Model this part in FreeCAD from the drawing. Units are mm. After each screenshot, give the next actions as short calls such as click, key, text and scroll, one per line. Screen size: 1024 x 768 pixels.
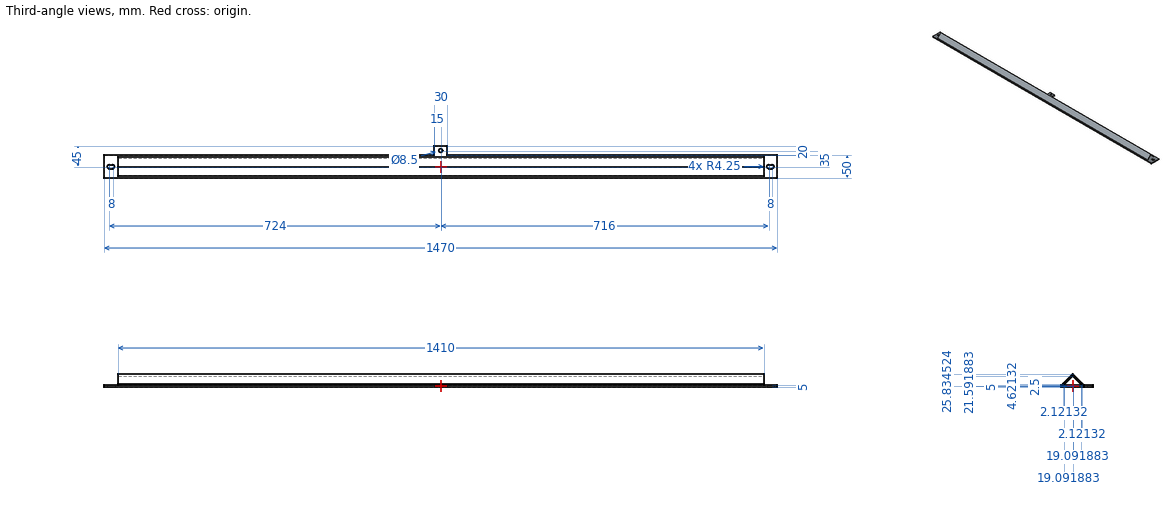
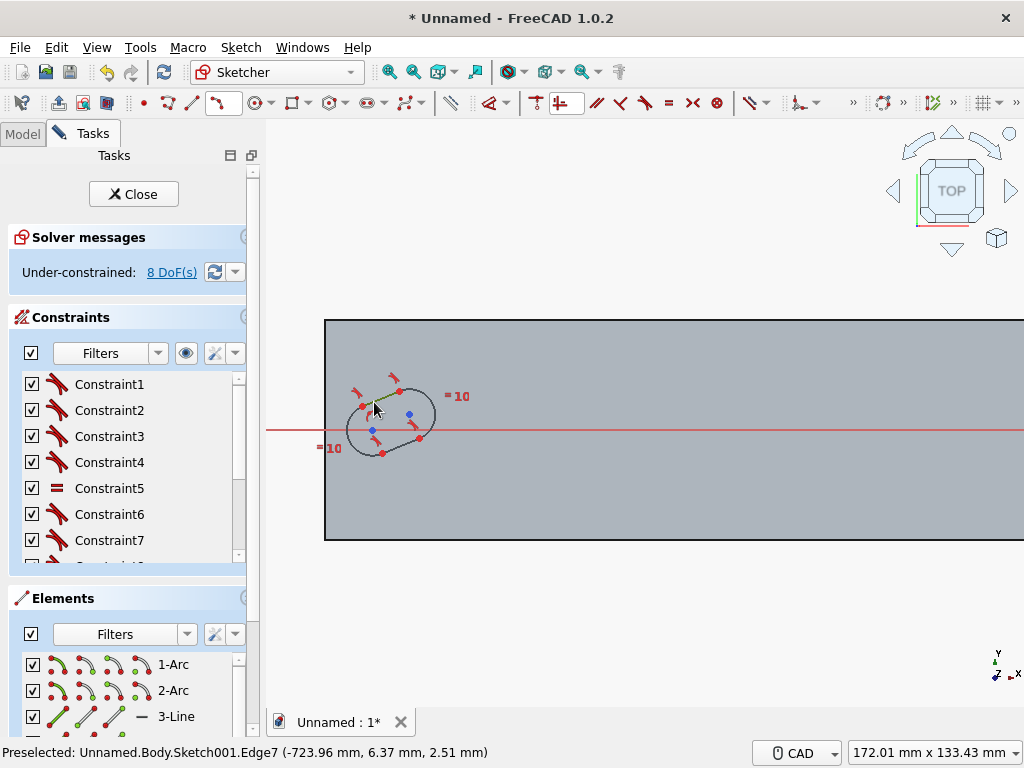
key(h)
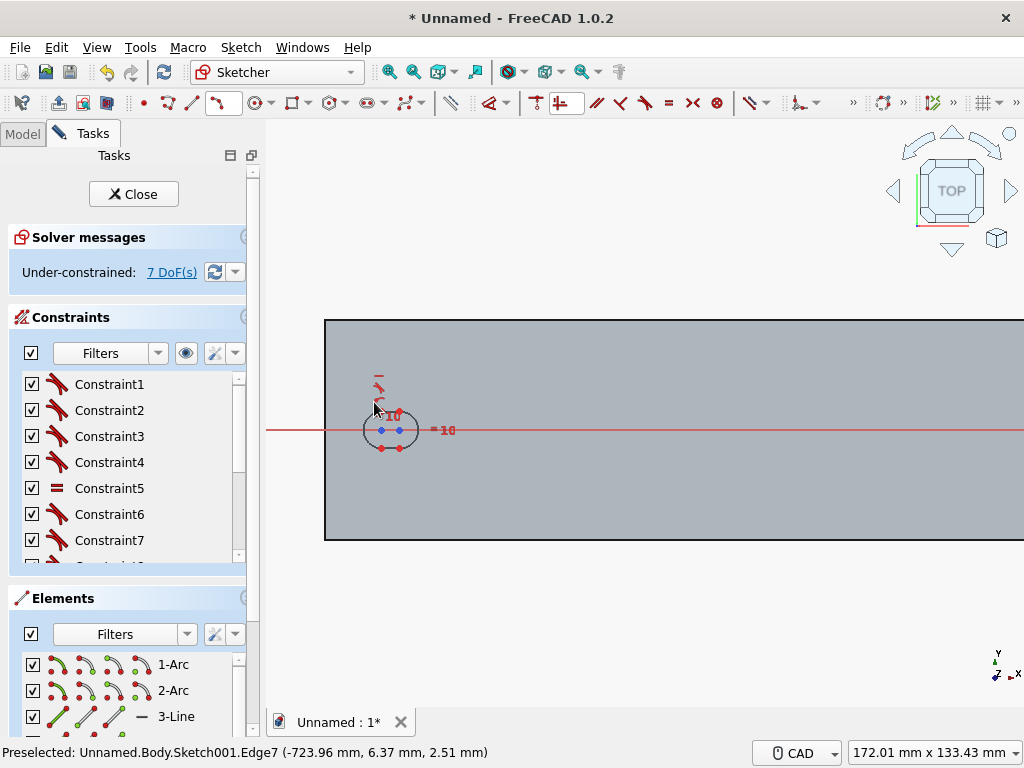
scroll(383, 412, down, 14)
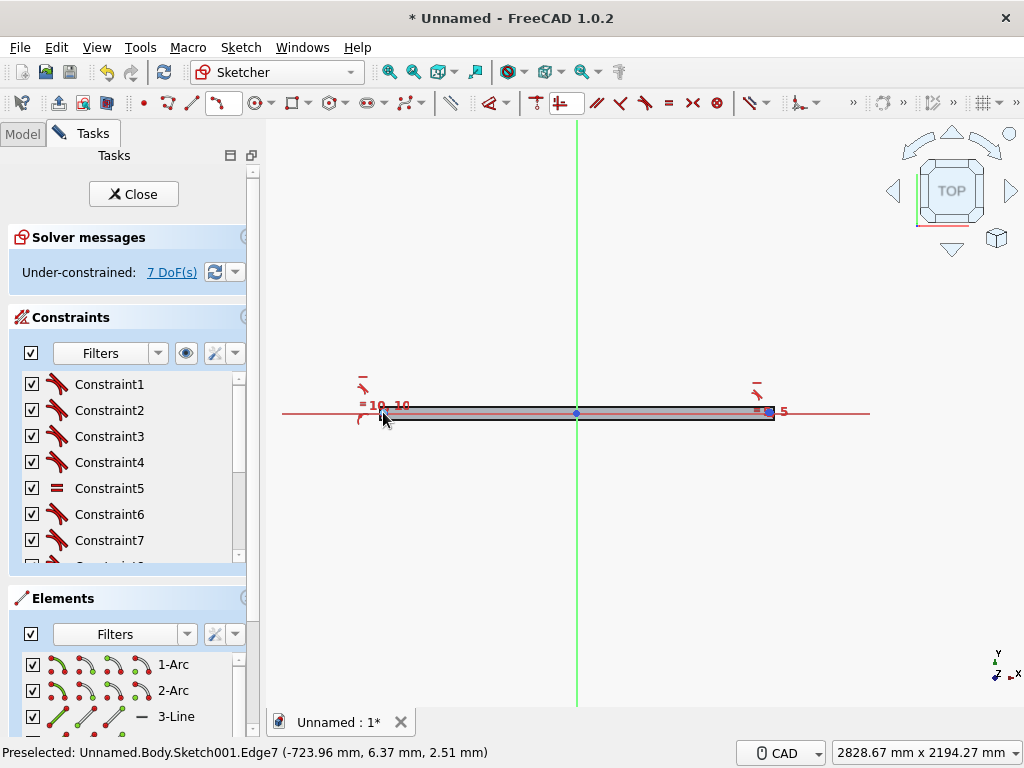
scroll(768, 413, up, 14)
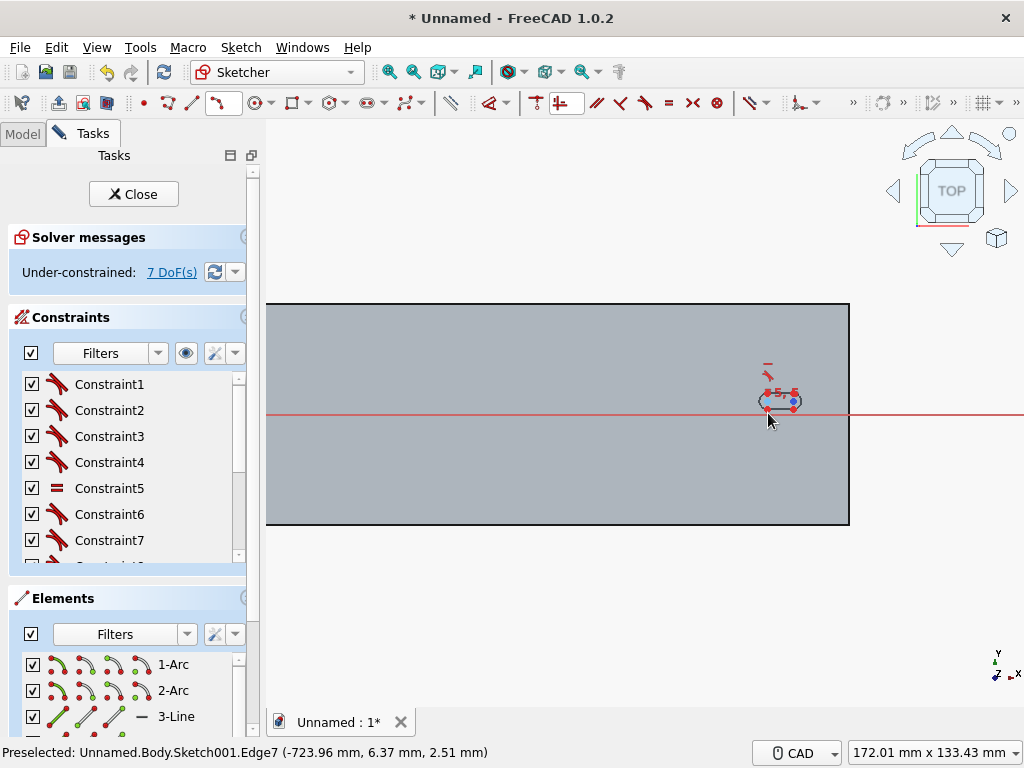
click(759, 401)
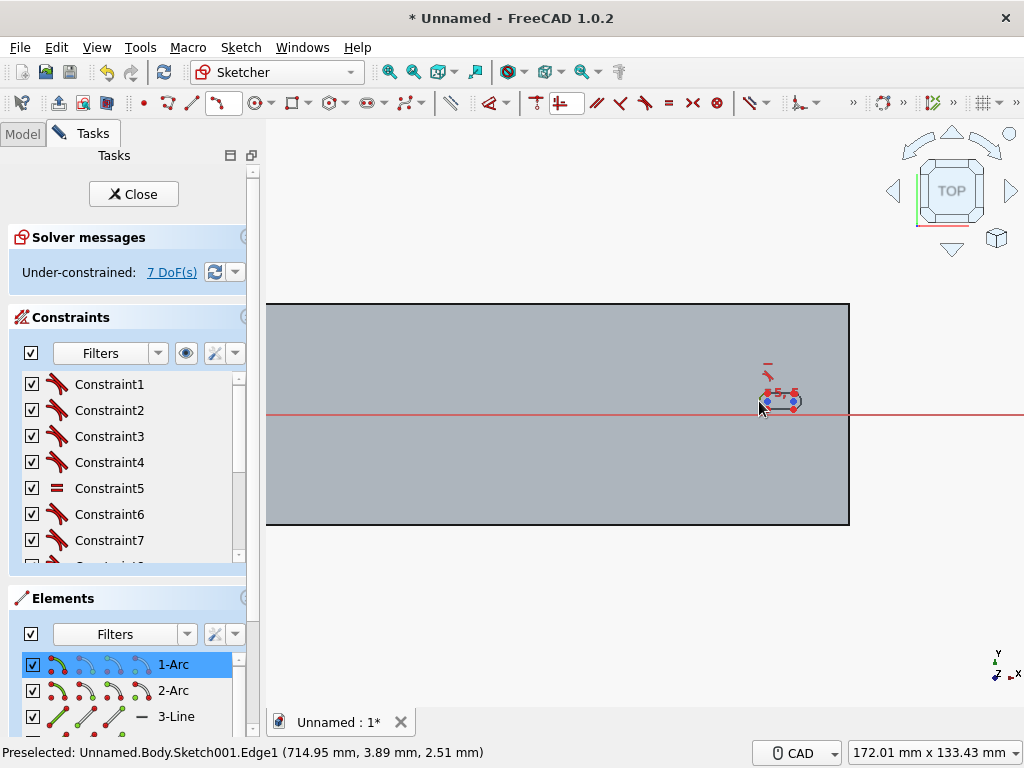
scroll(769, 413, down, 14)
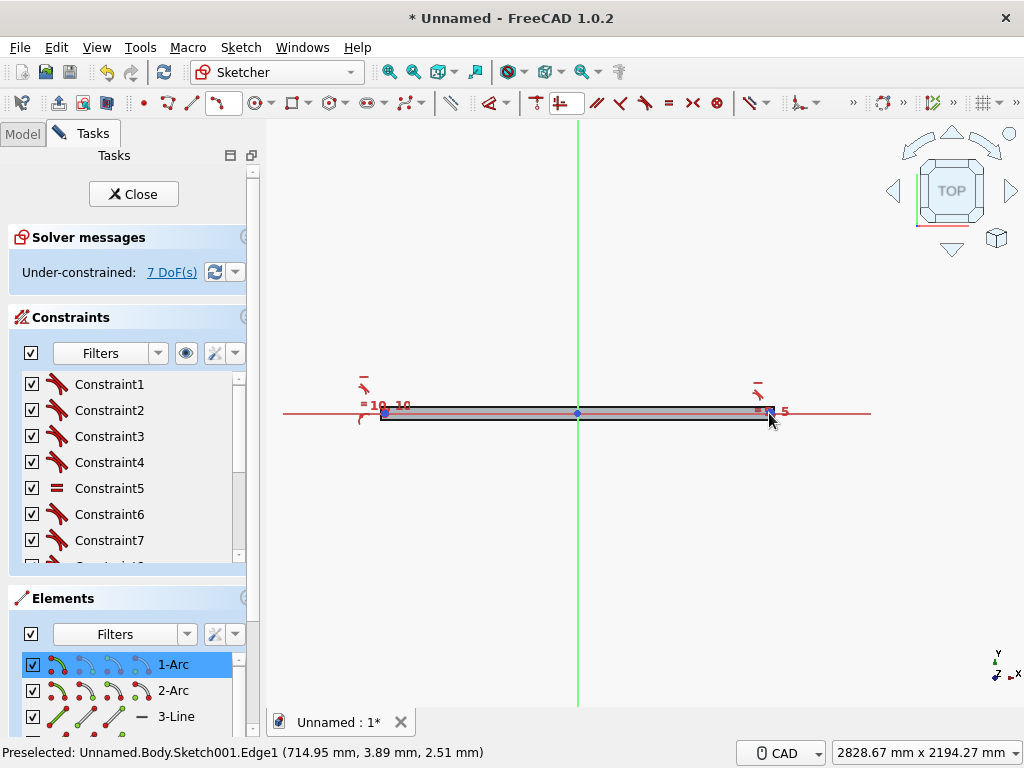
scroll(383, 413, up, 14)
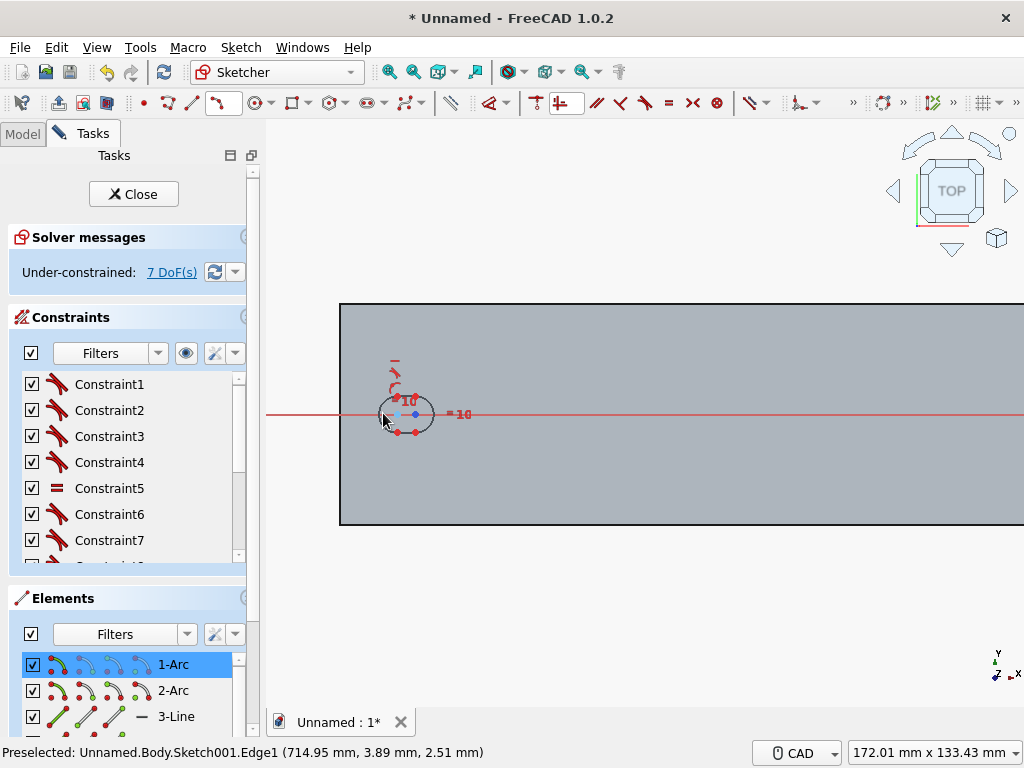
click(383, 404)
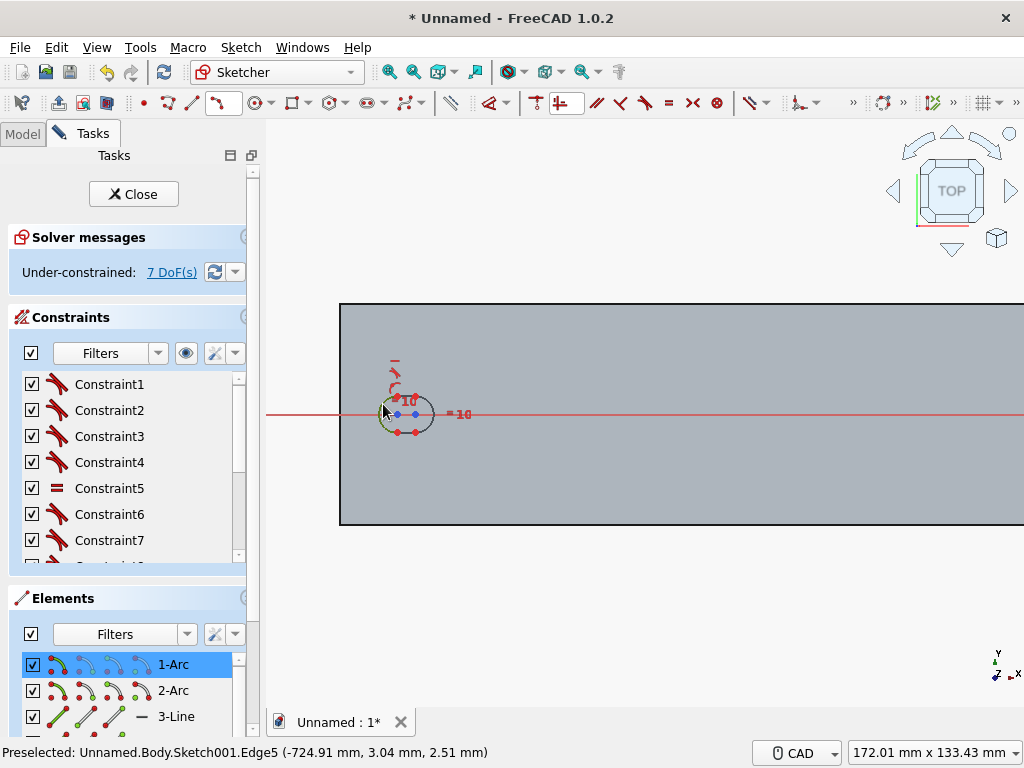
click(670, 104)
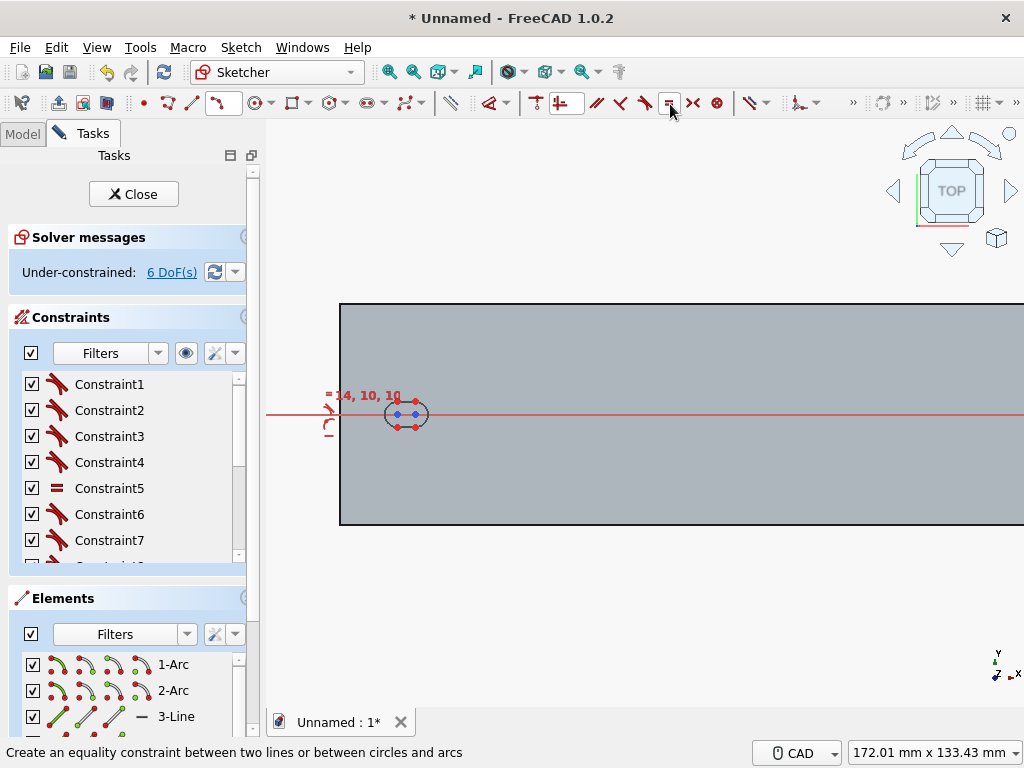
scroll(382, 413, down, 14)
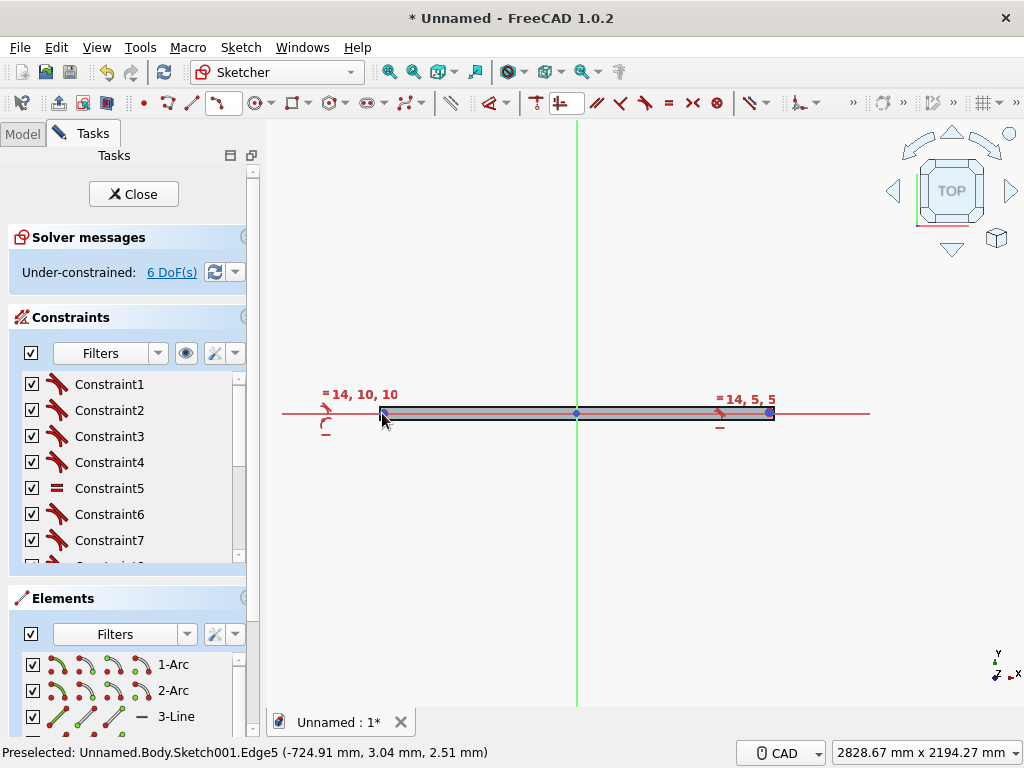
scroll(769, 413, up, 14)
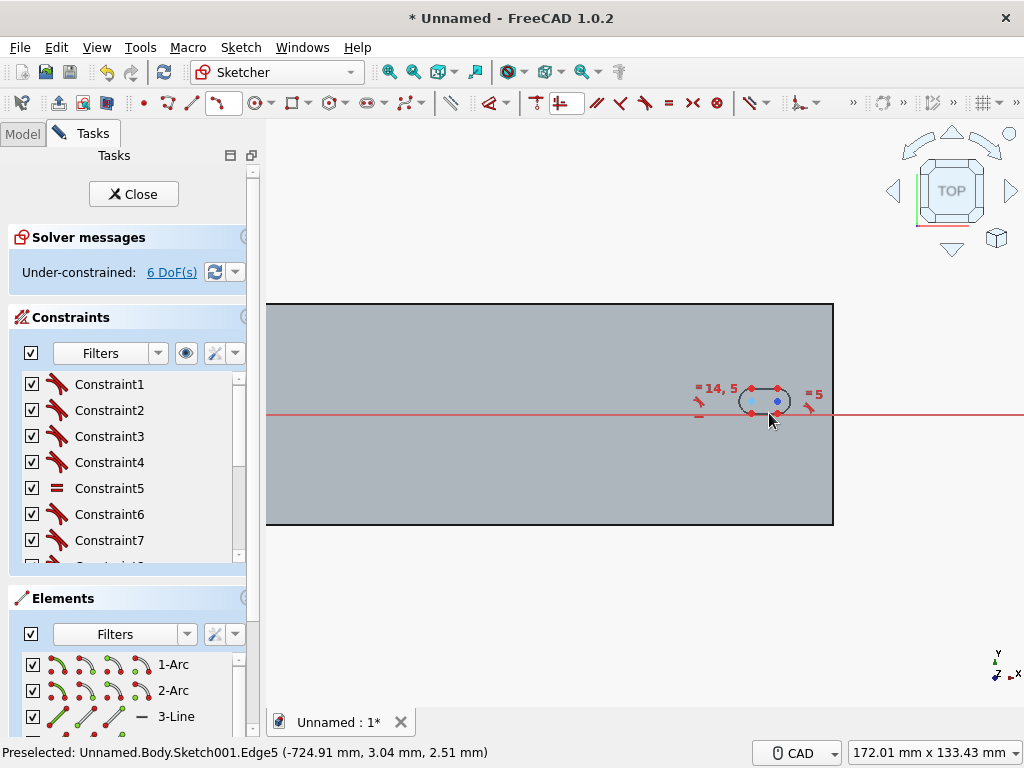
click(752, 401)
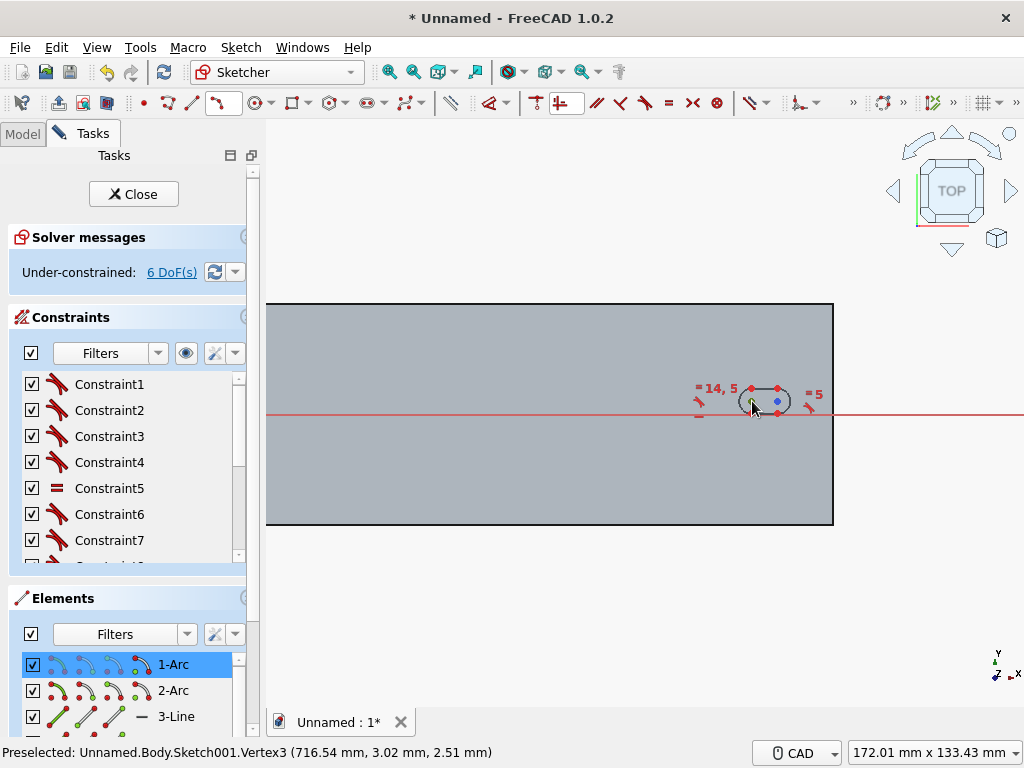
click(334, 415)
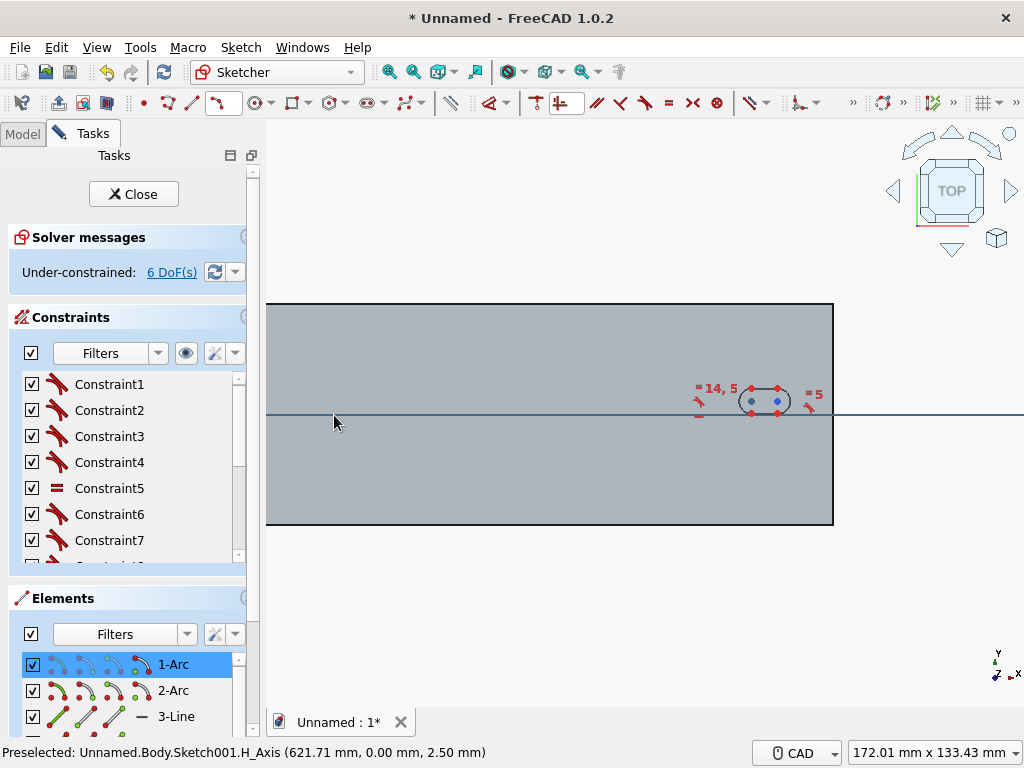
click(536, 104)